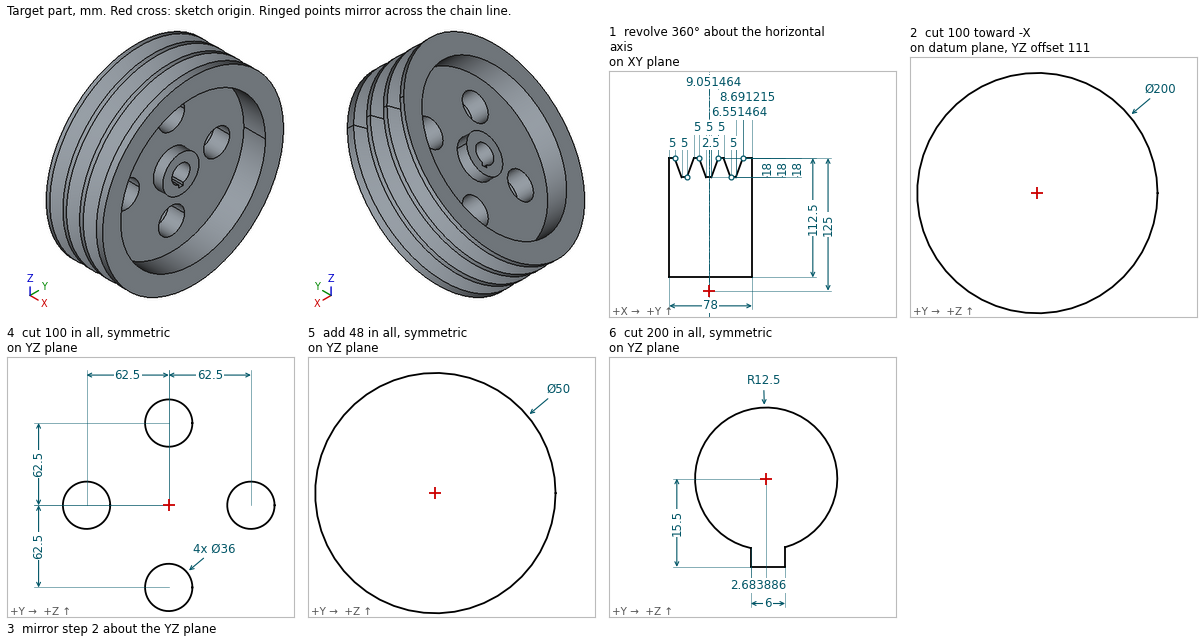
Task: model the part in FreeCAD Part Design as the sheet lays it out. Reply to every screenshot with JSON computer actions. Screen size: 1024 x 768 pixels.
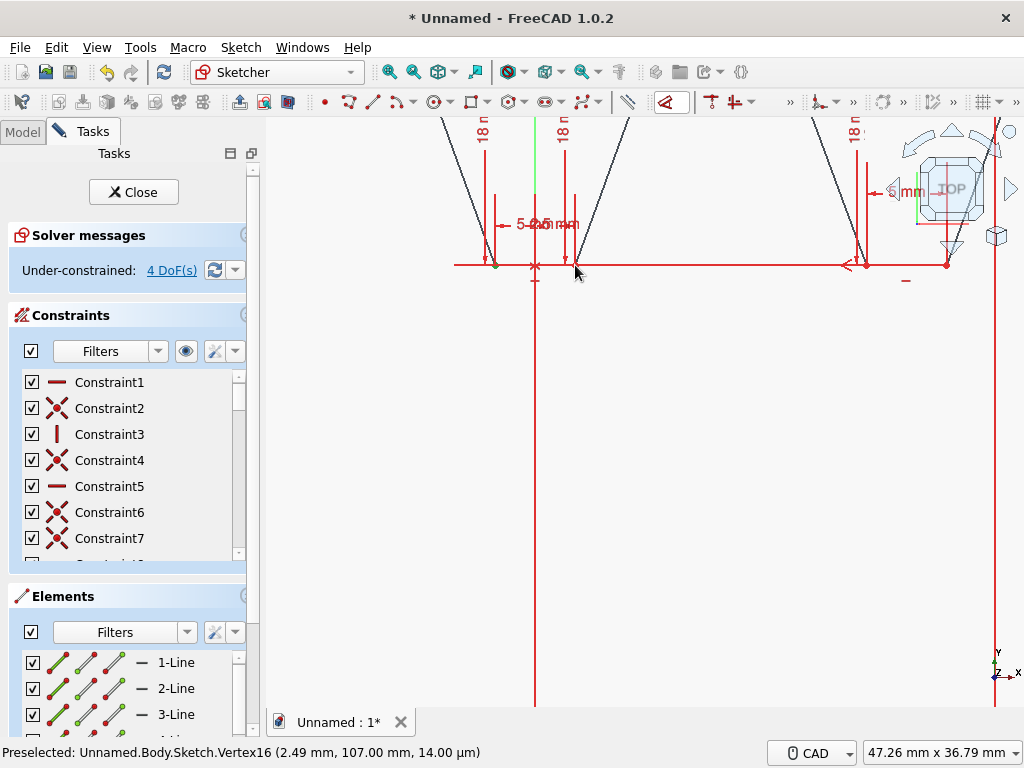
{"action": "scroll", "coordinate": [579, 269], "scroll_direction": "down", "scroll_amount": 8}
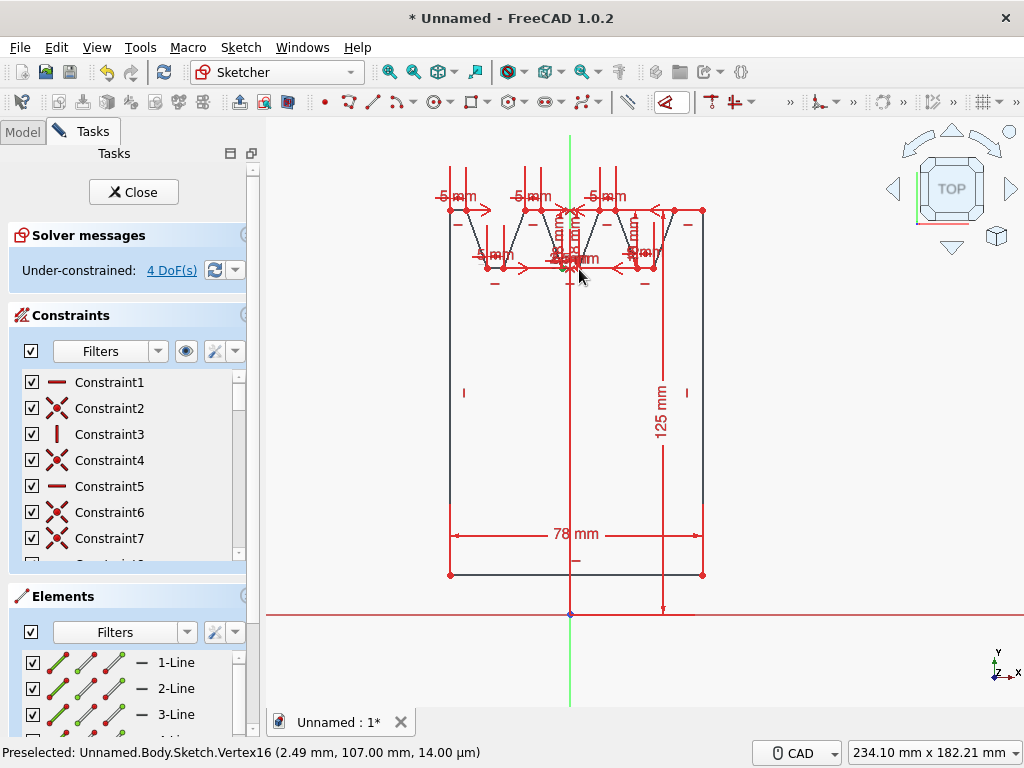
{"action": "left_click", "coordinate": [703, 466]}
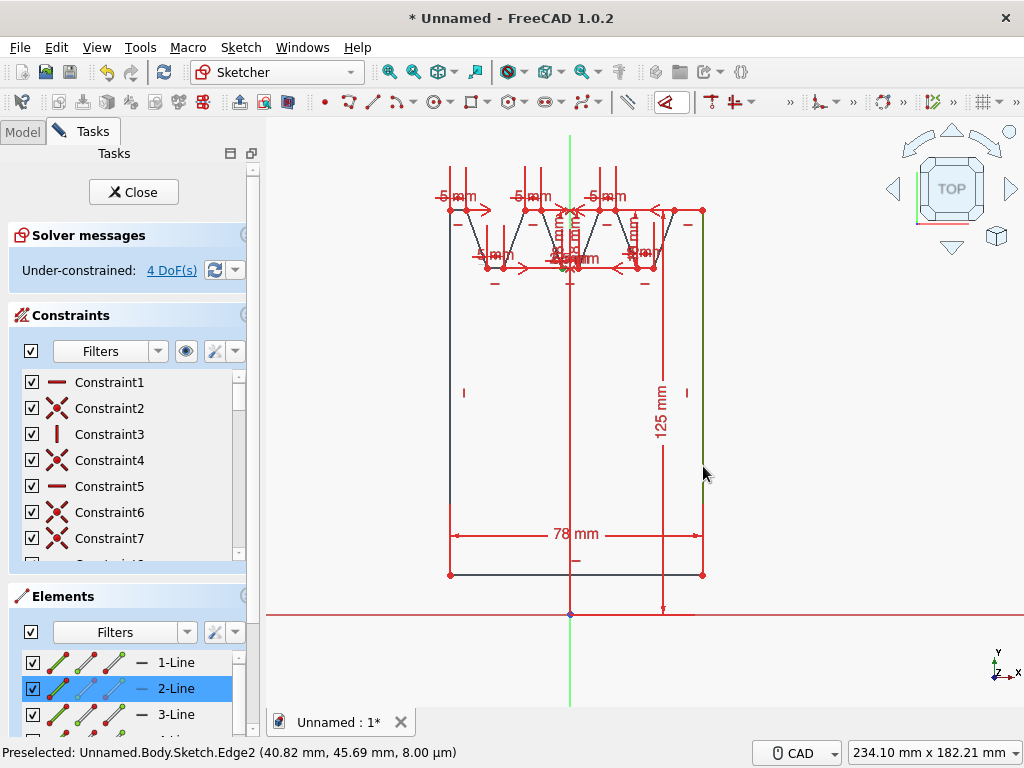
{"action": "key", "text": "i"}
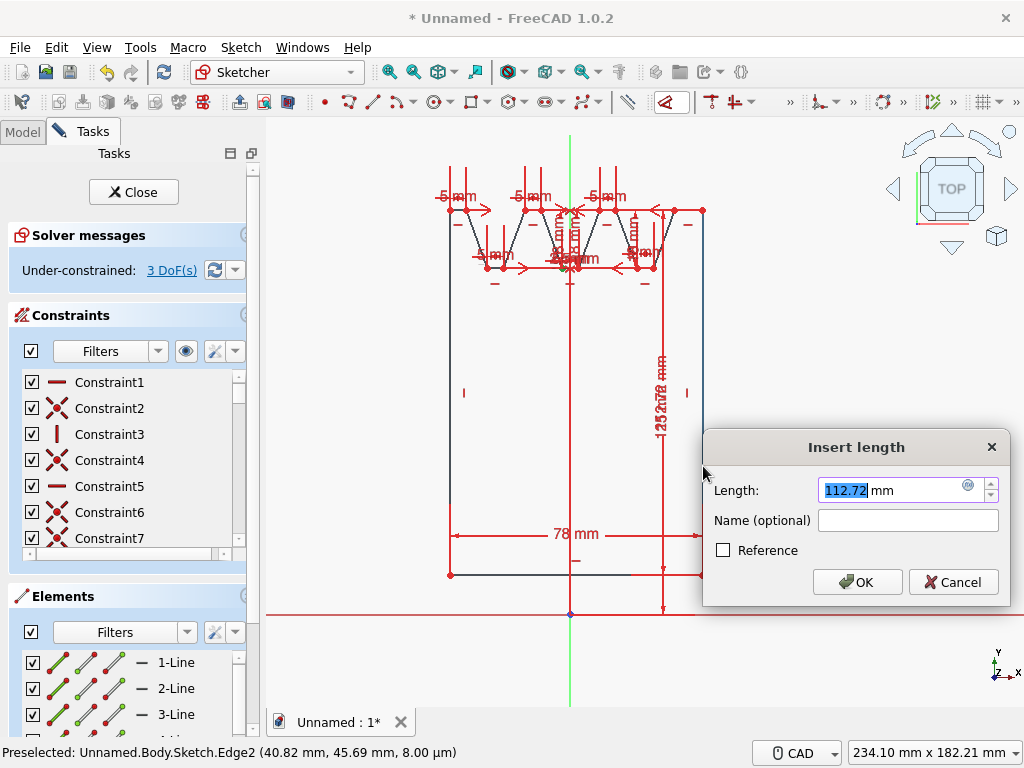
{"action": "type", "text": "112.5"}
{"action": "key", "text": "Return"}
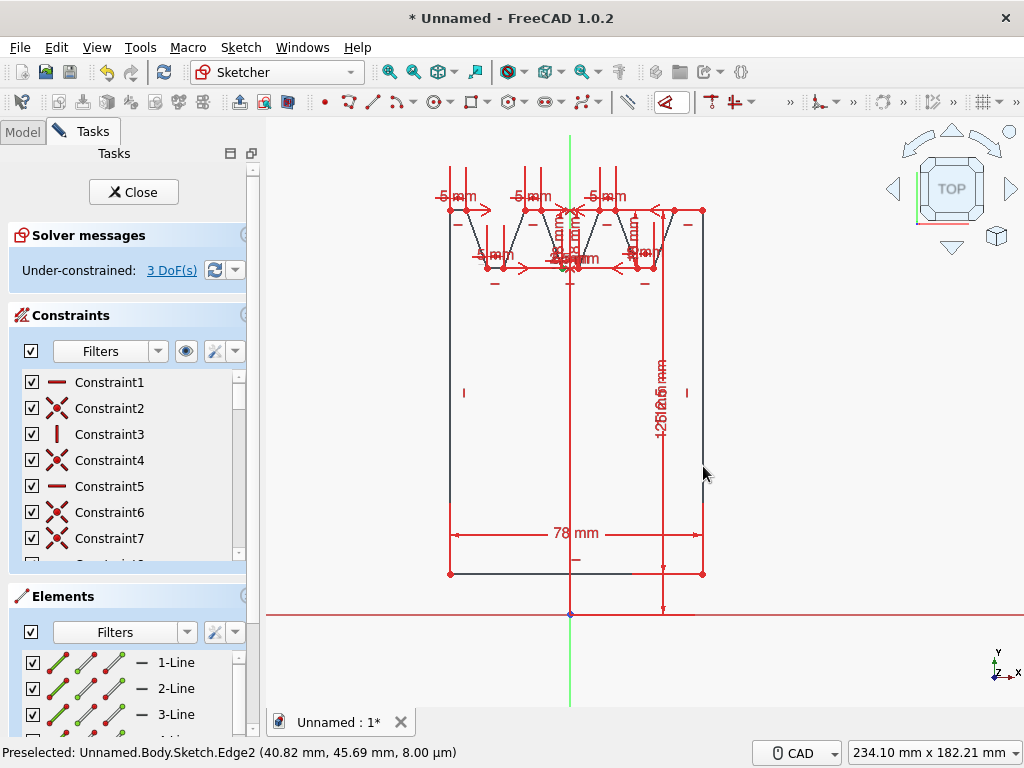
{"action": "scroll", "coordinate": [691, 210], "scroll_direction": "up", "scroll_amount": 2}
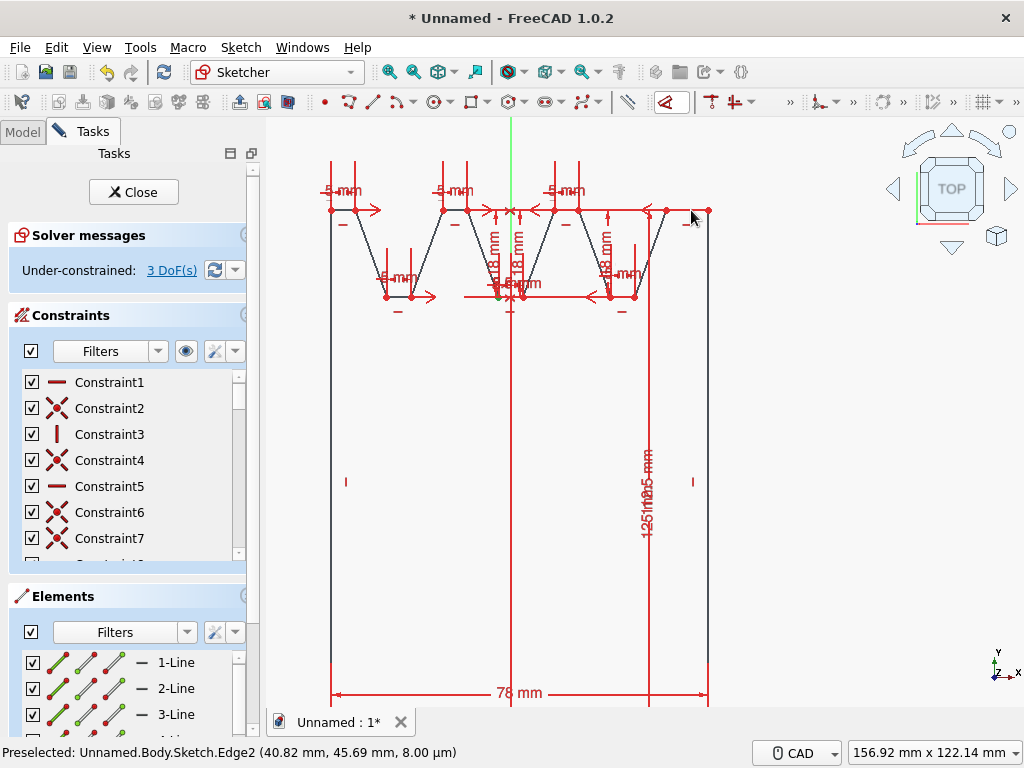
{"action": "left_click", "coordinate": [691, 210]}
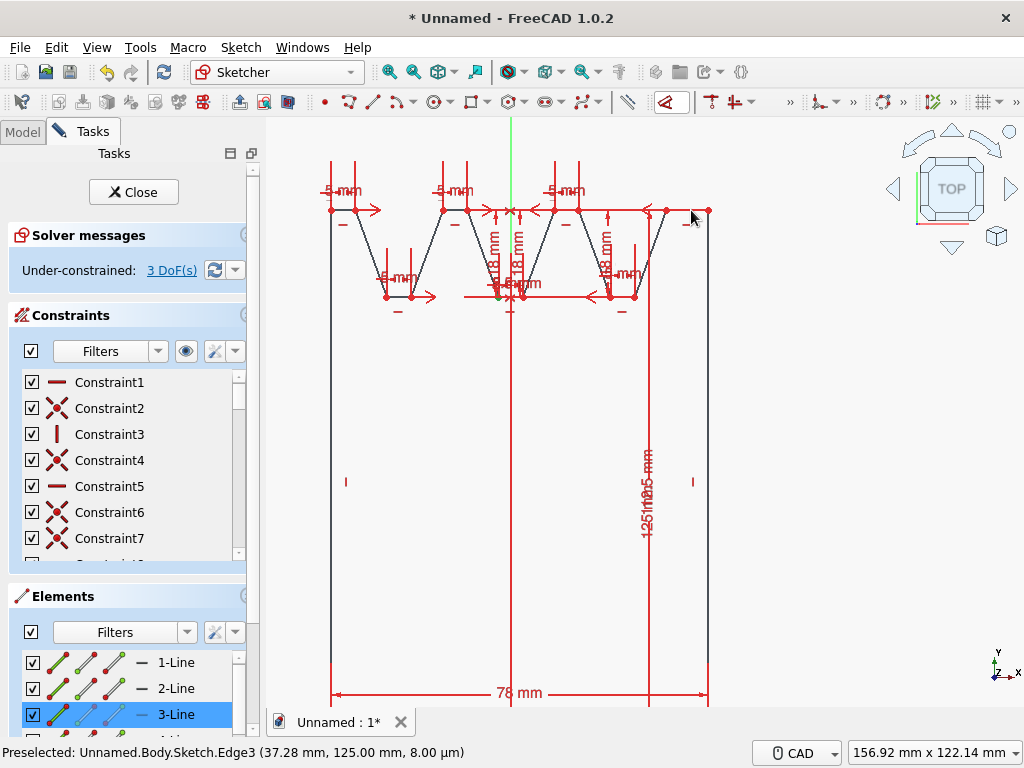
{"action": "key", "text": "l"}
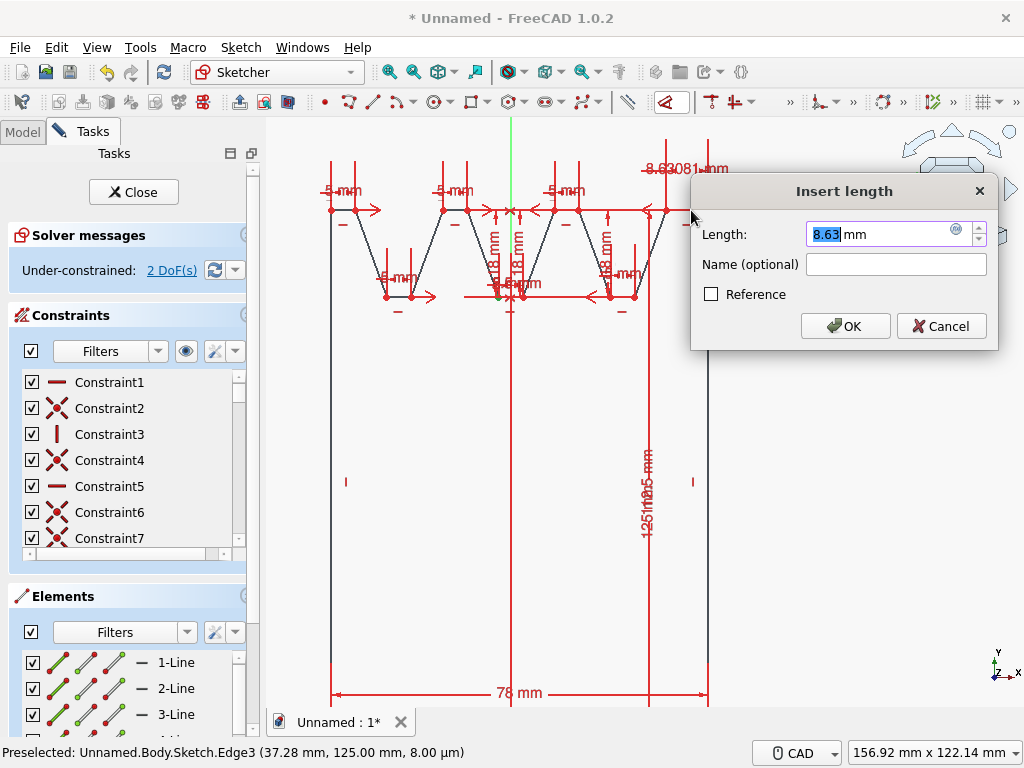
{"action": "type", "text": "8.691215"}
{"action": "key", "text": "Return"}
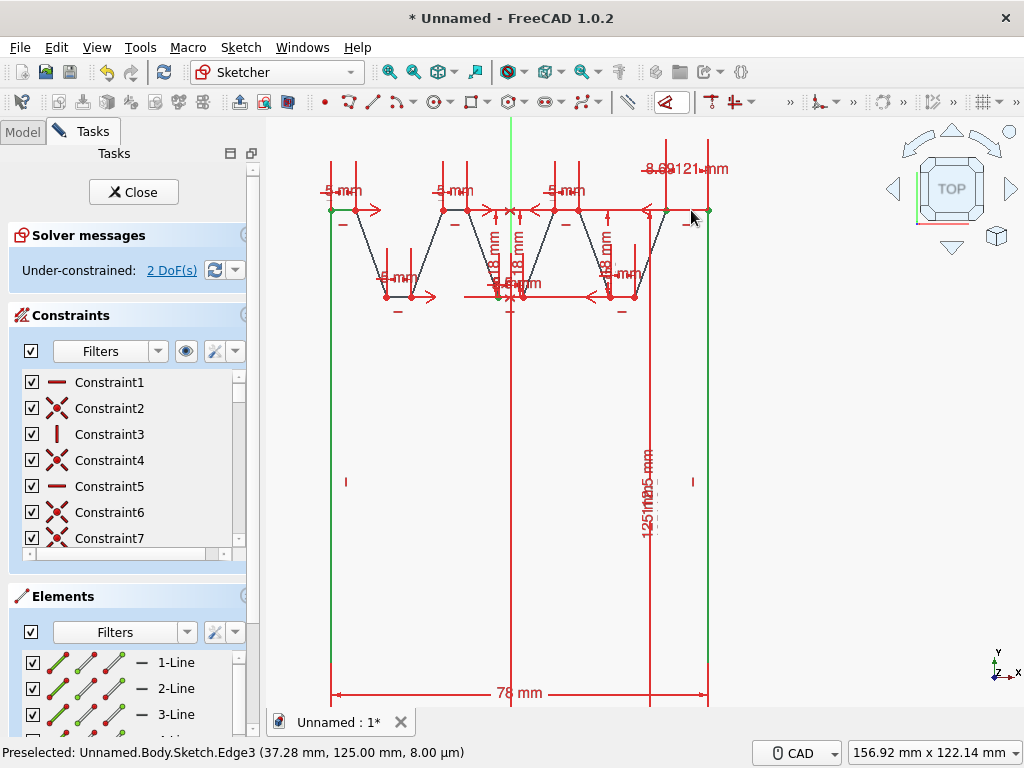
{"action": "left_click", "coordinate": [555, 210]}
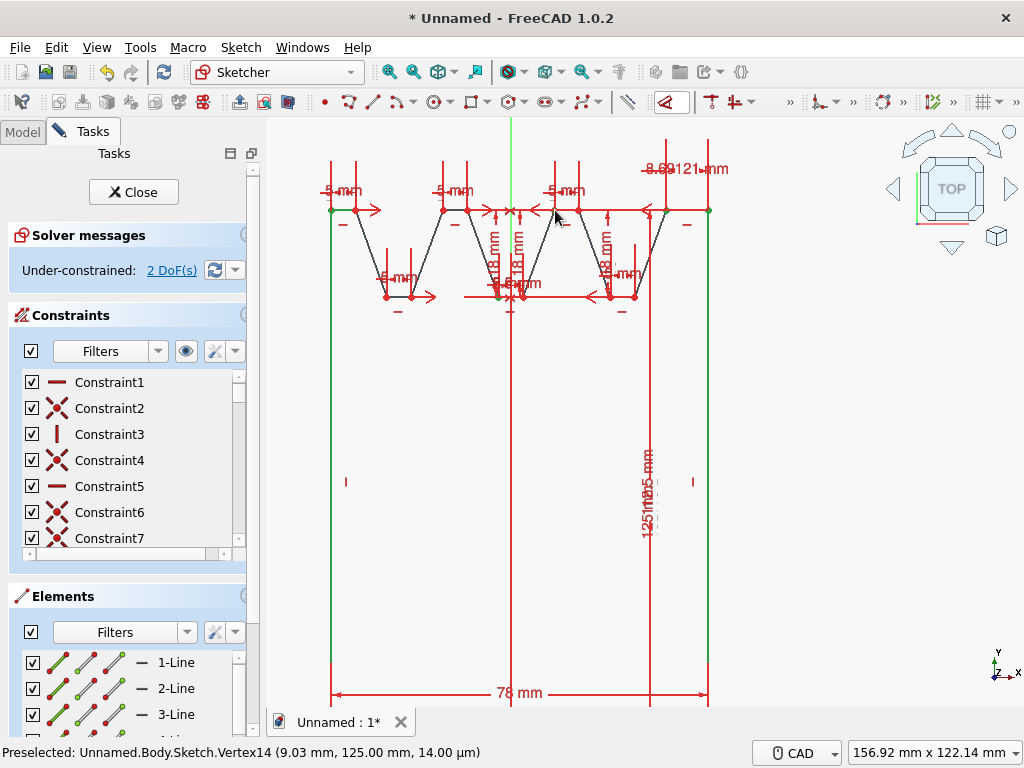
{"action": "key", "text": "l"}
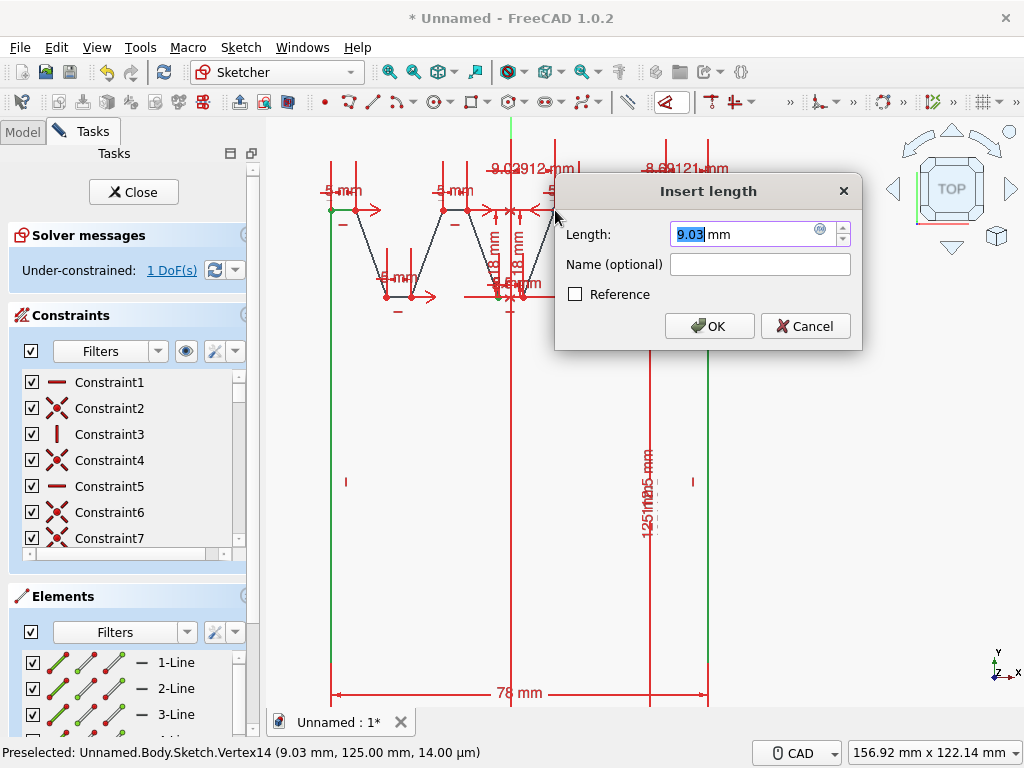
{"action": "type", "text": "9.051464"}
{"action": "key", "text": "Return"}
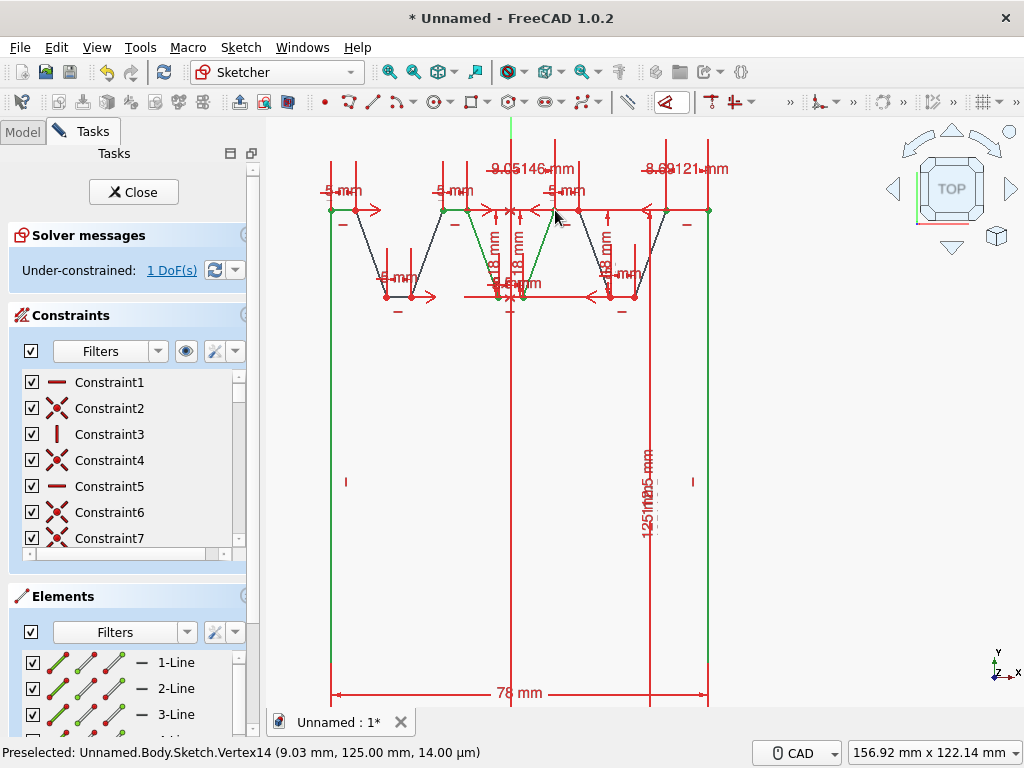
{"action": "scroll", "coordinate": [657, 236], "scroll_direction": "up", "scroll_amount": 2}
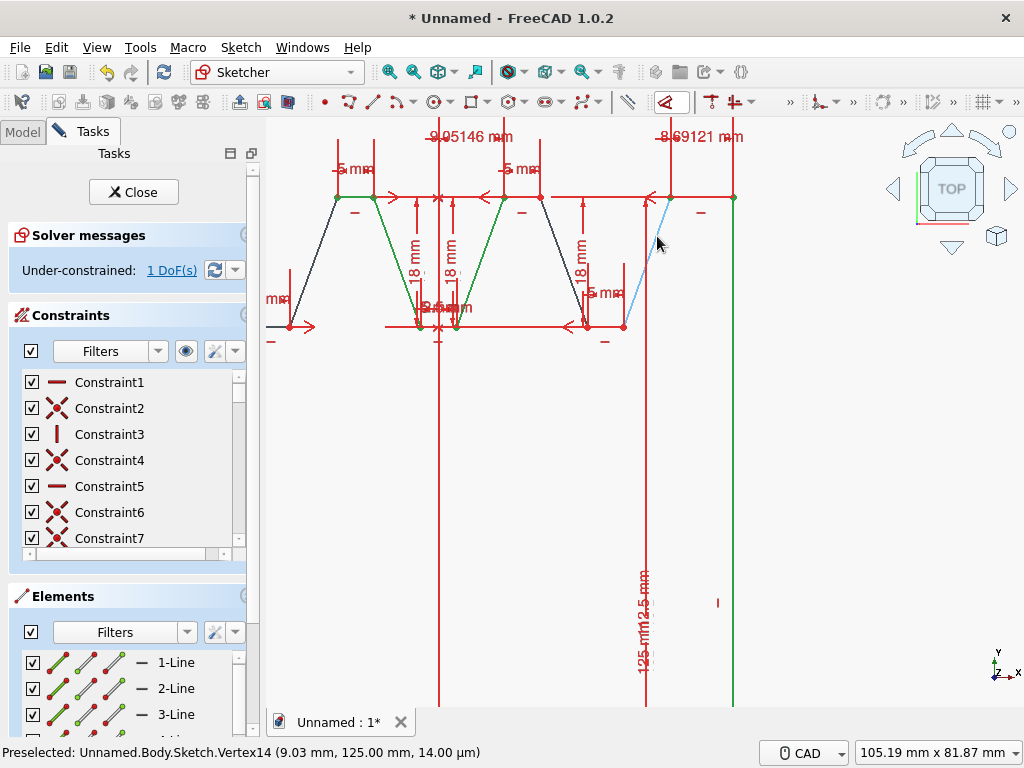
{"action": "left_click", "coordinate": [657, 236]}